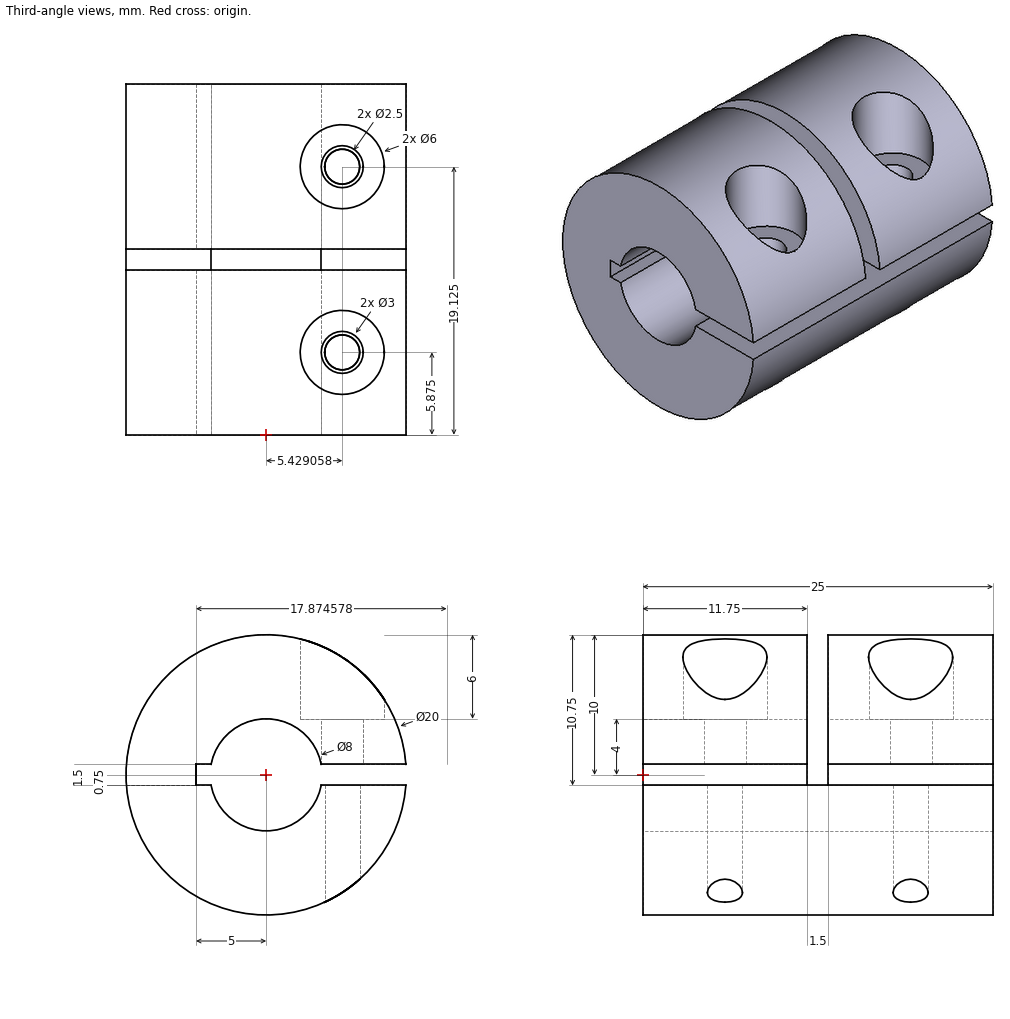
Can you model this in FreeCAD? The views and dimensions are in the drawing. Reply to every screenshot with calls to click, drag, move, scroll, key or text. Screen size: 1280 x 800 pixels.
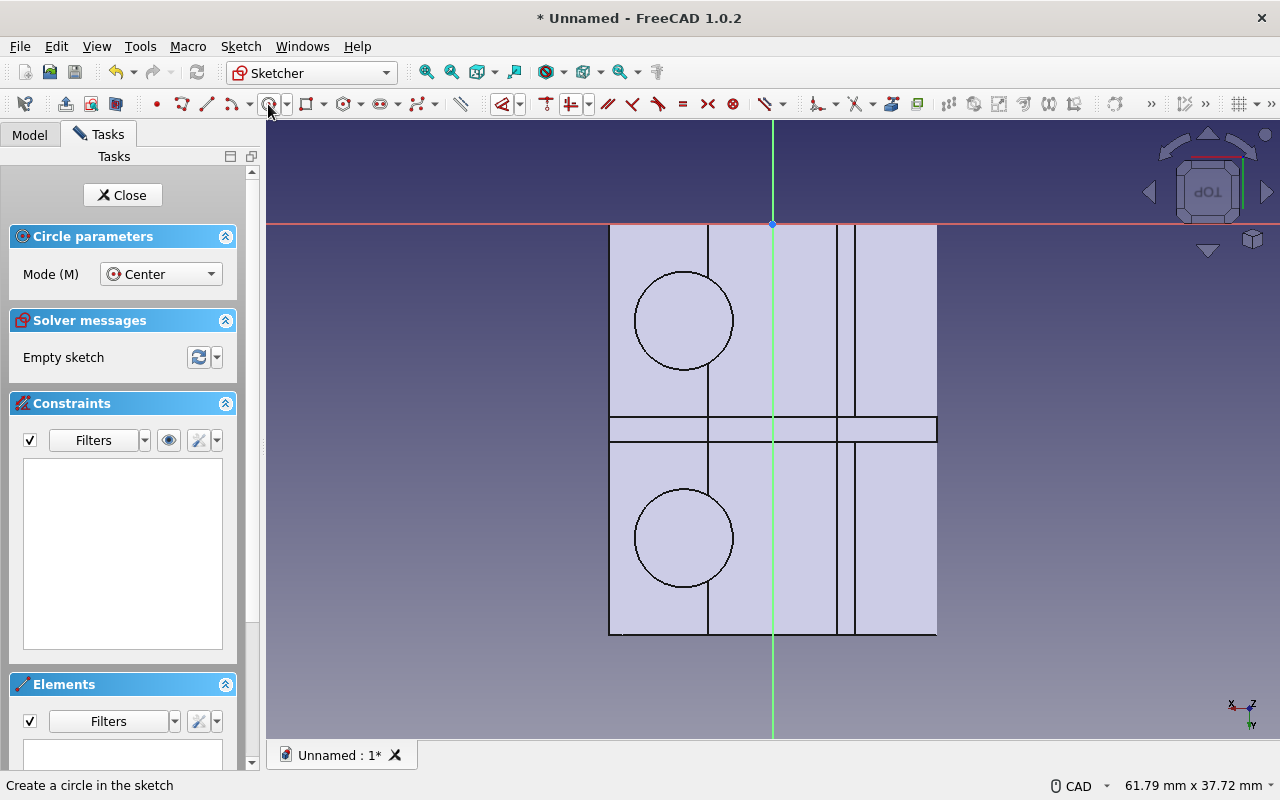
click(684, 321)
click(701, 303)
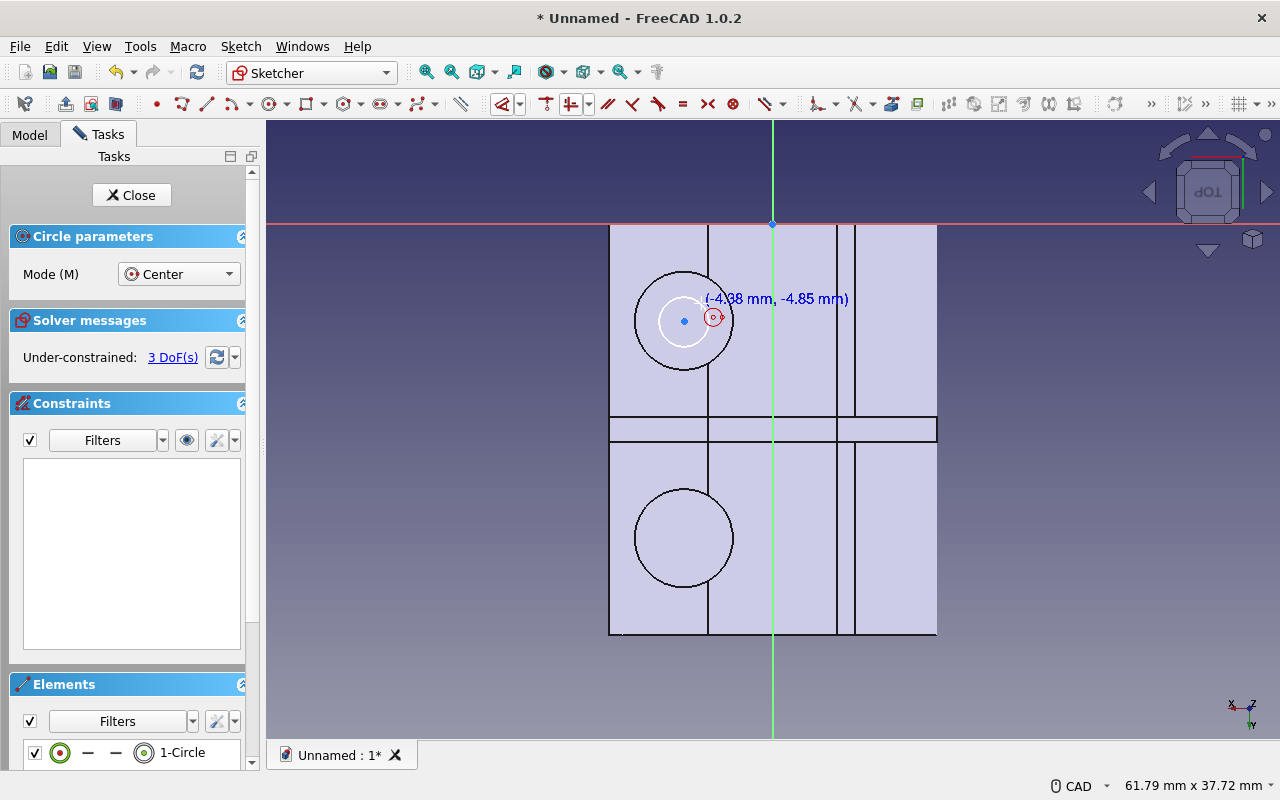
click(684, 538)
click(701, 521)
key(Escape)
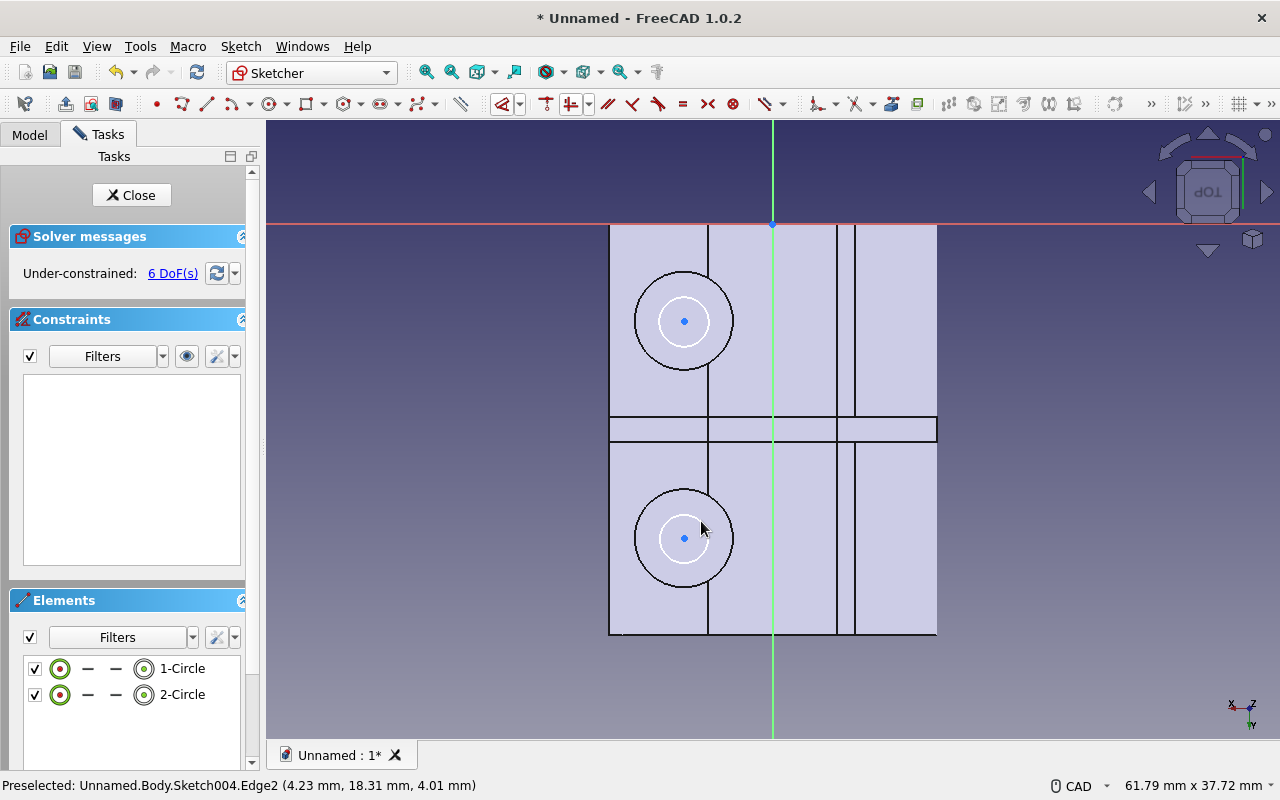
click(701, 304)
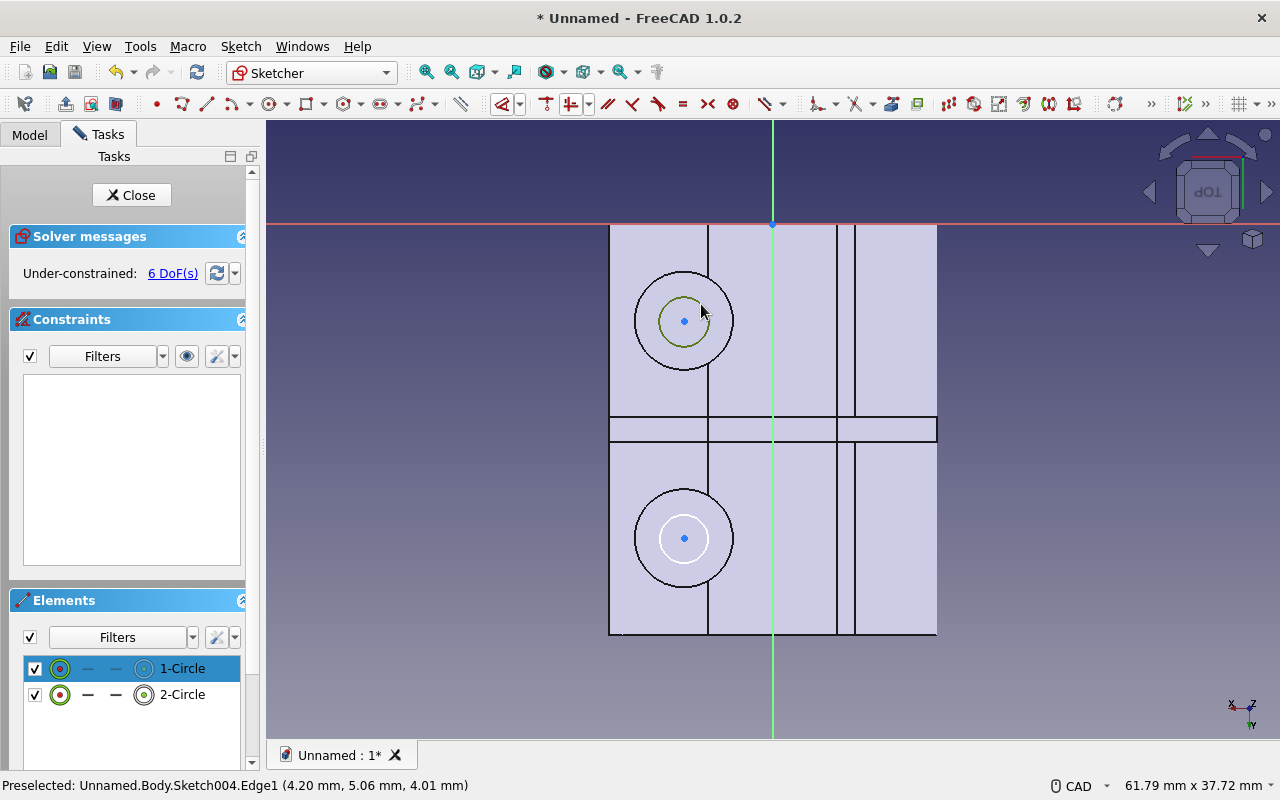
click(701, 522)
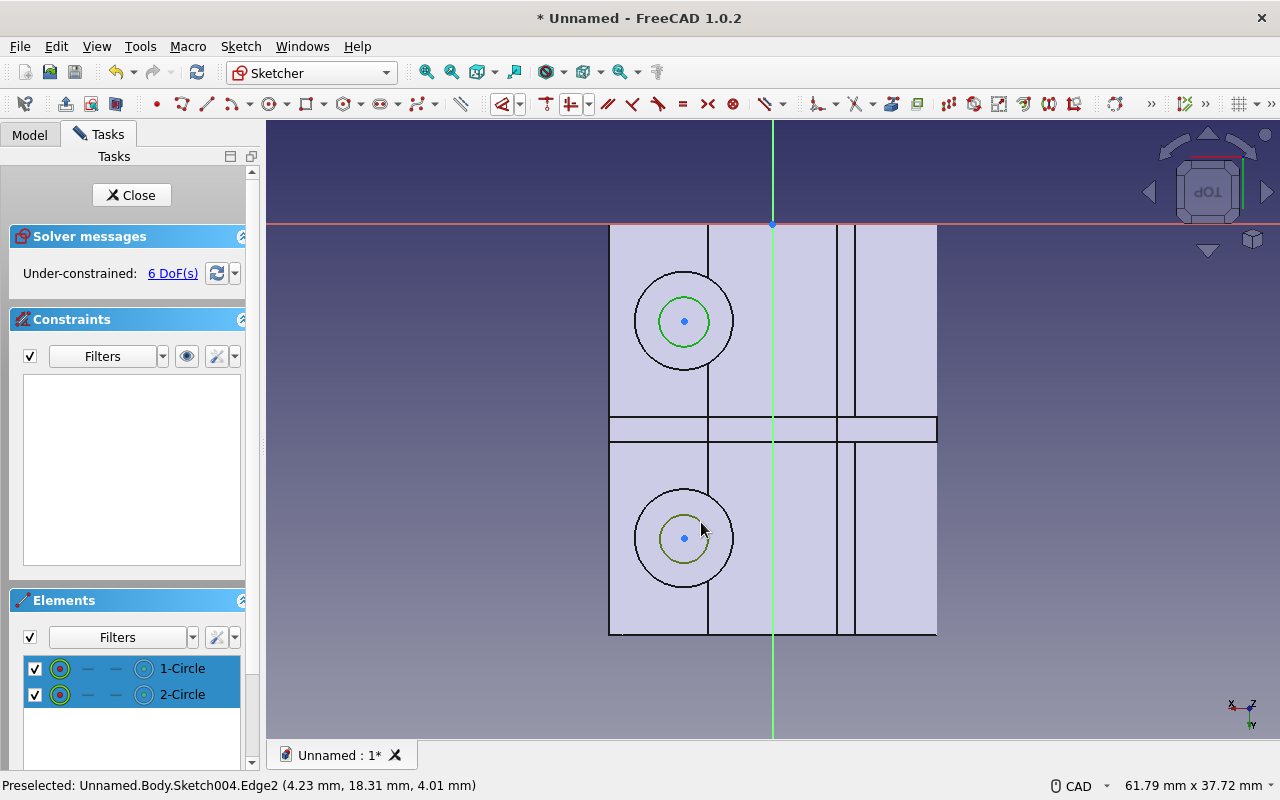
click(683, 104)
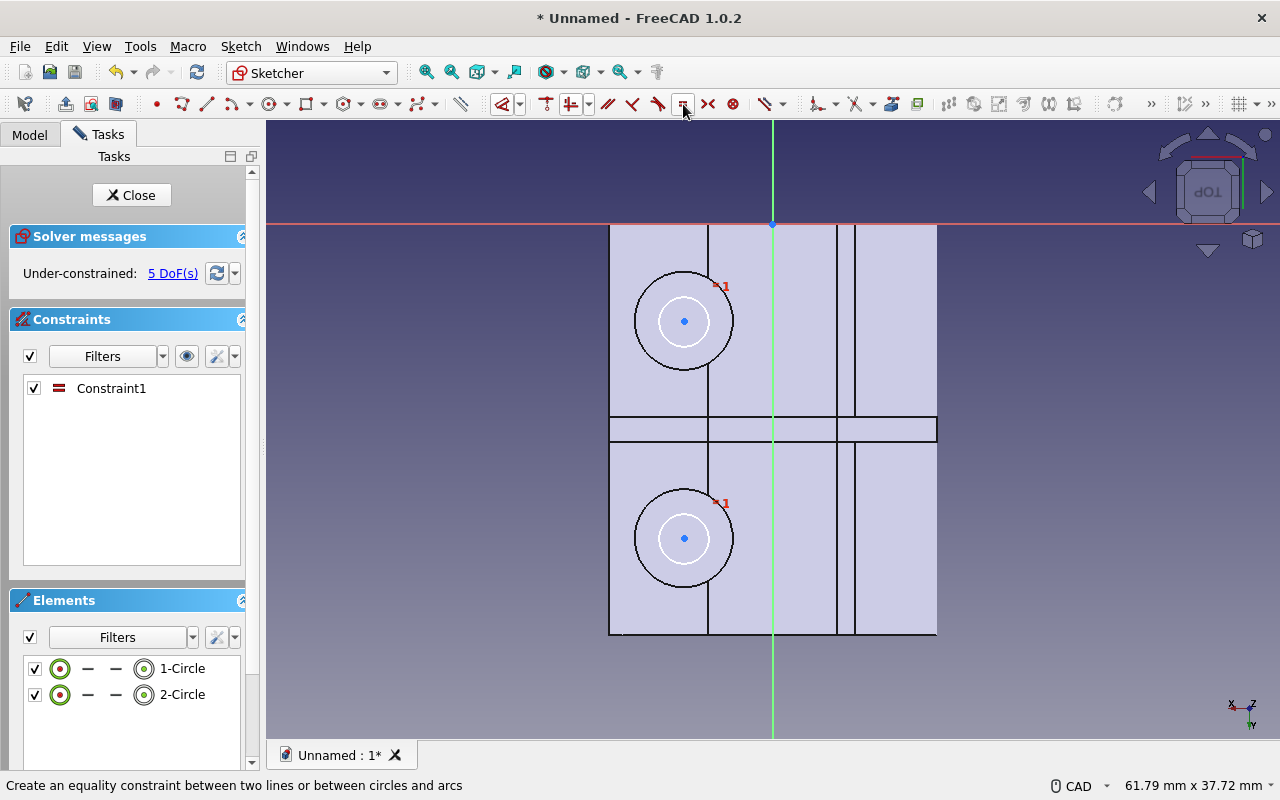
click(684, 322)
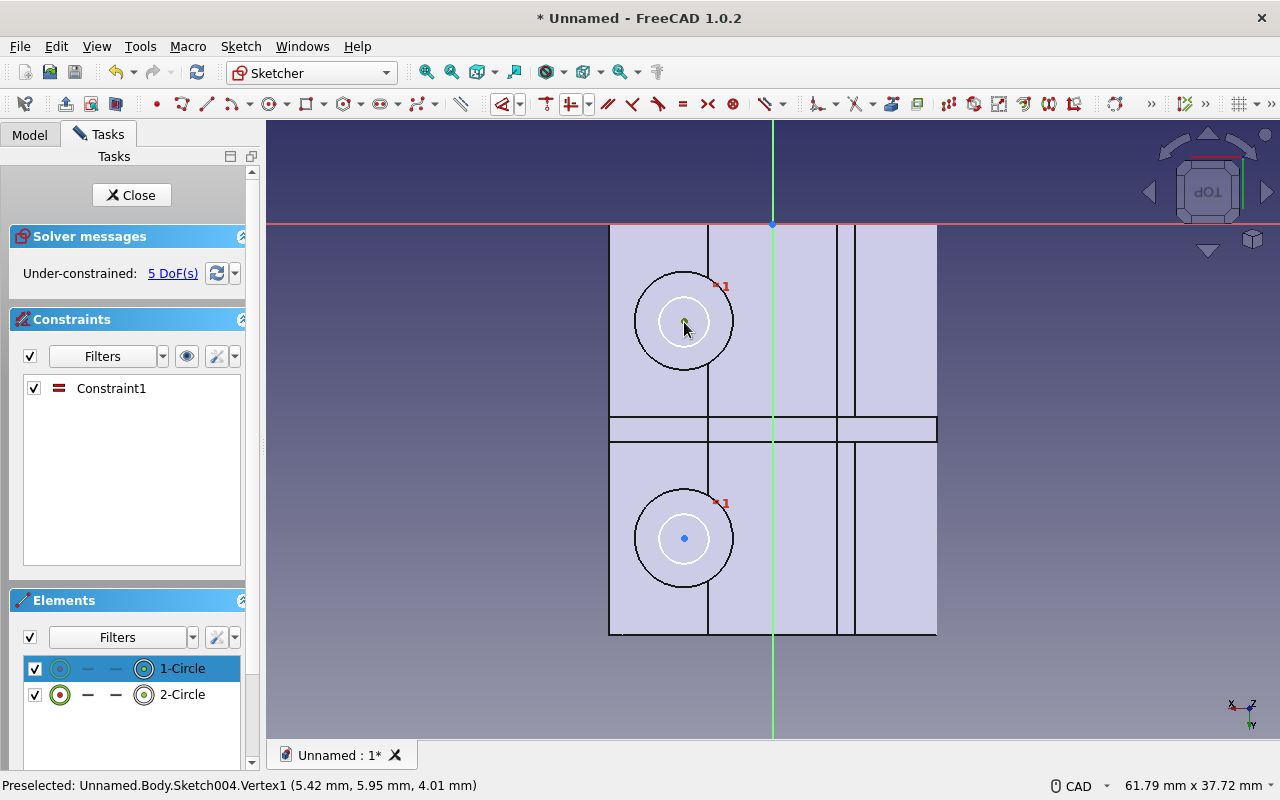
click(684, 539)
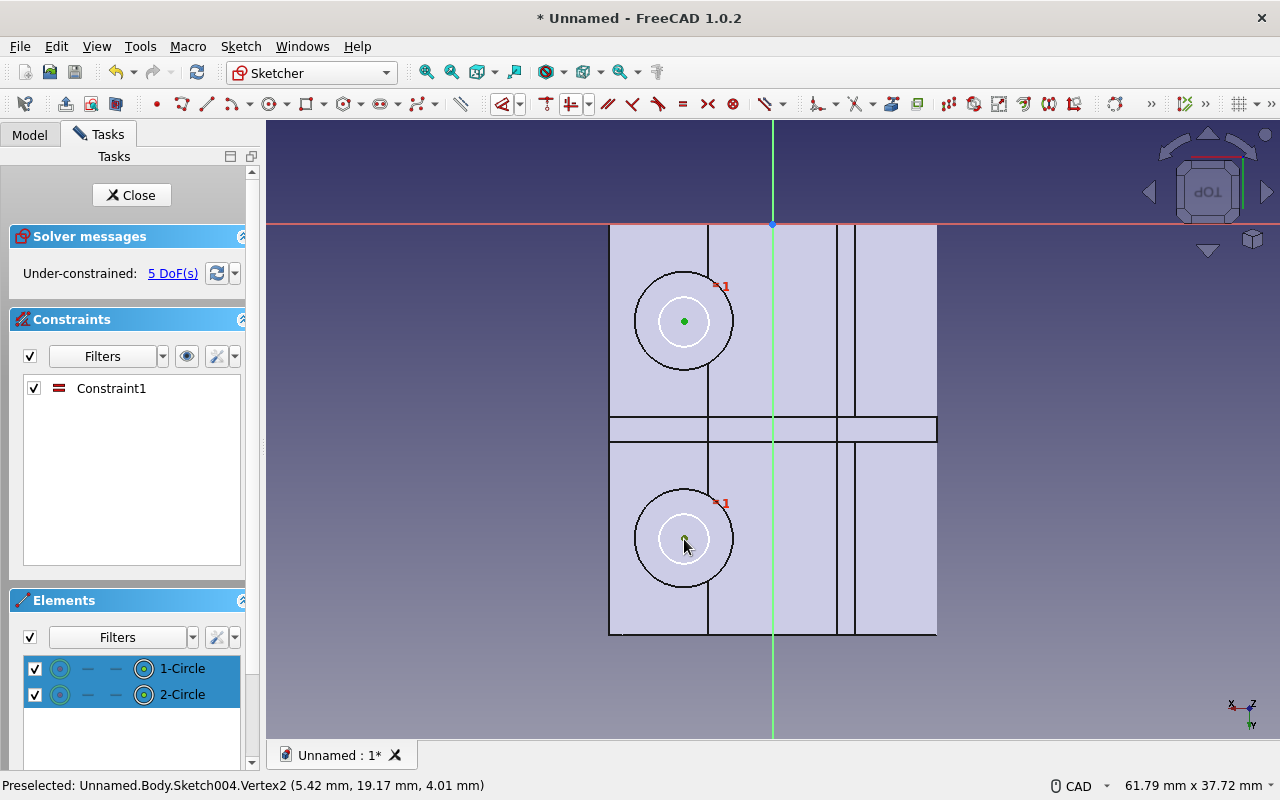
click(588, 104)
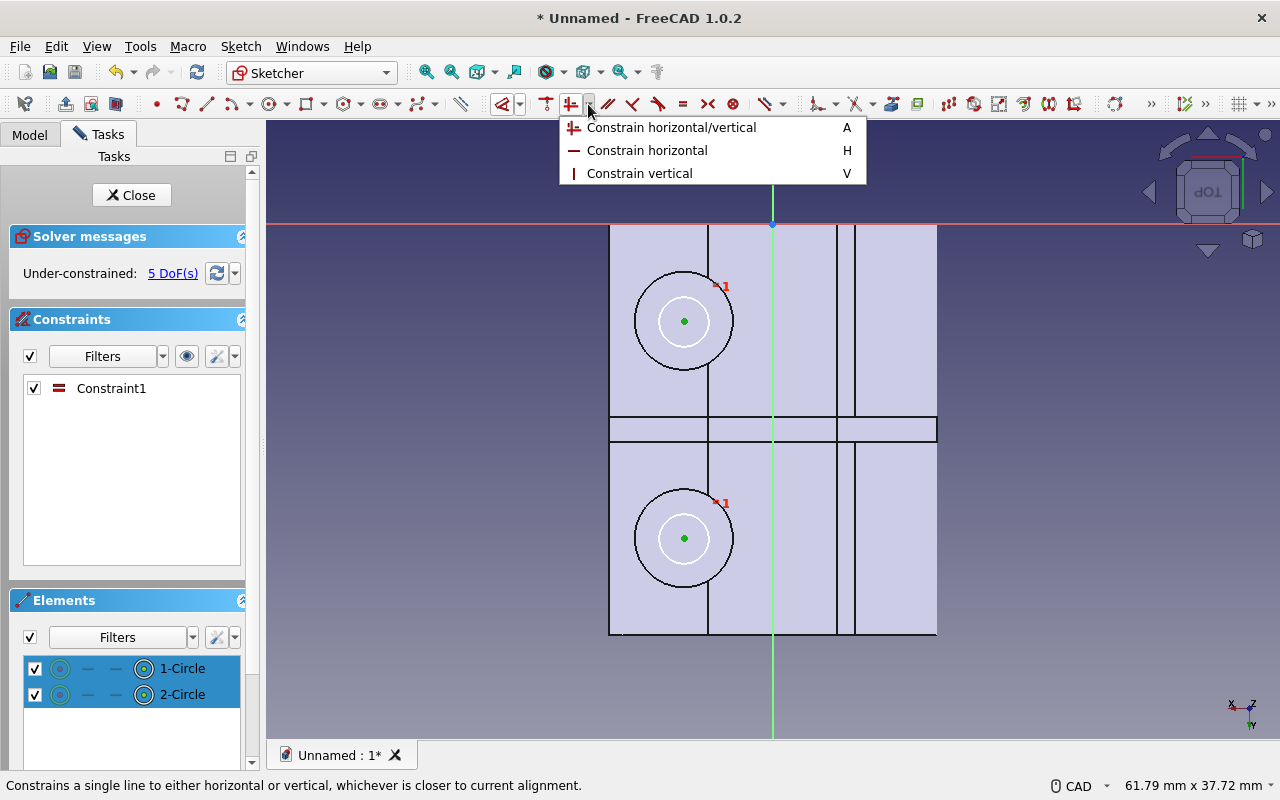
click(713, 174)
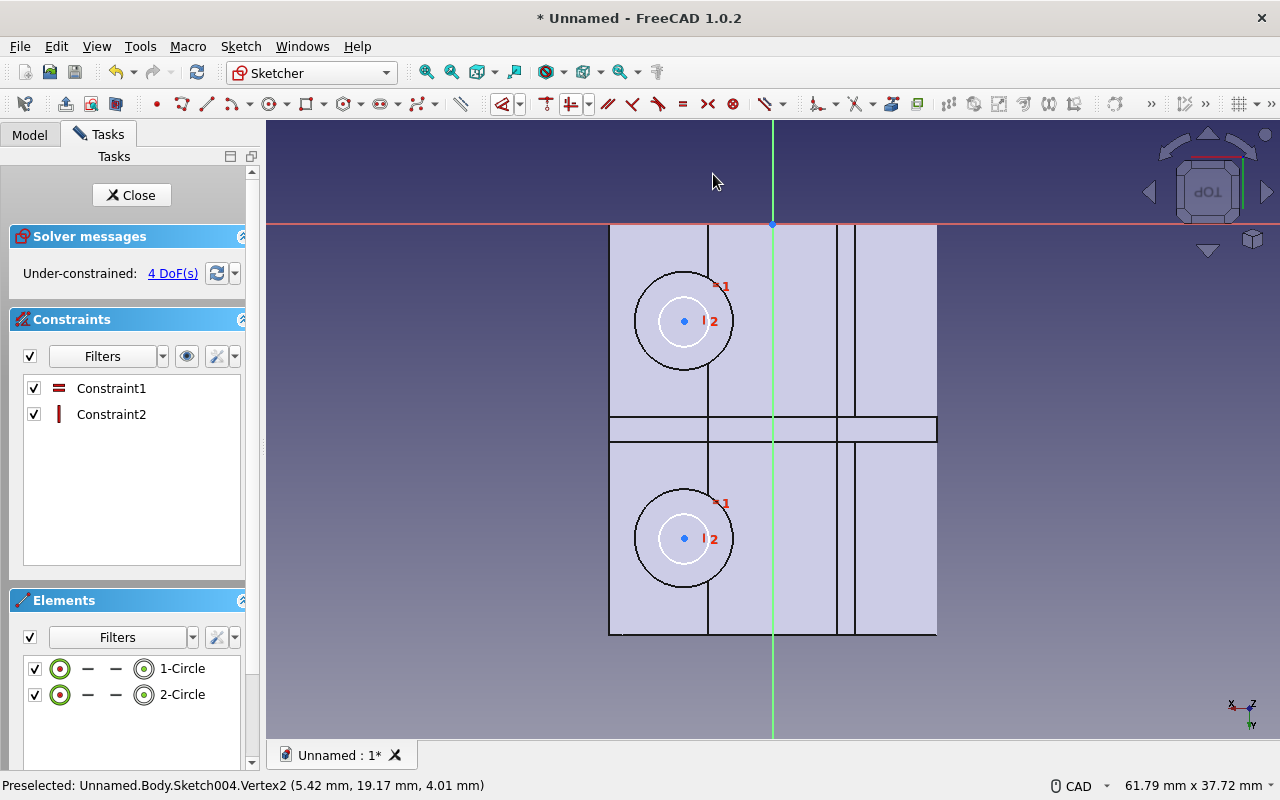
click(701, 304)